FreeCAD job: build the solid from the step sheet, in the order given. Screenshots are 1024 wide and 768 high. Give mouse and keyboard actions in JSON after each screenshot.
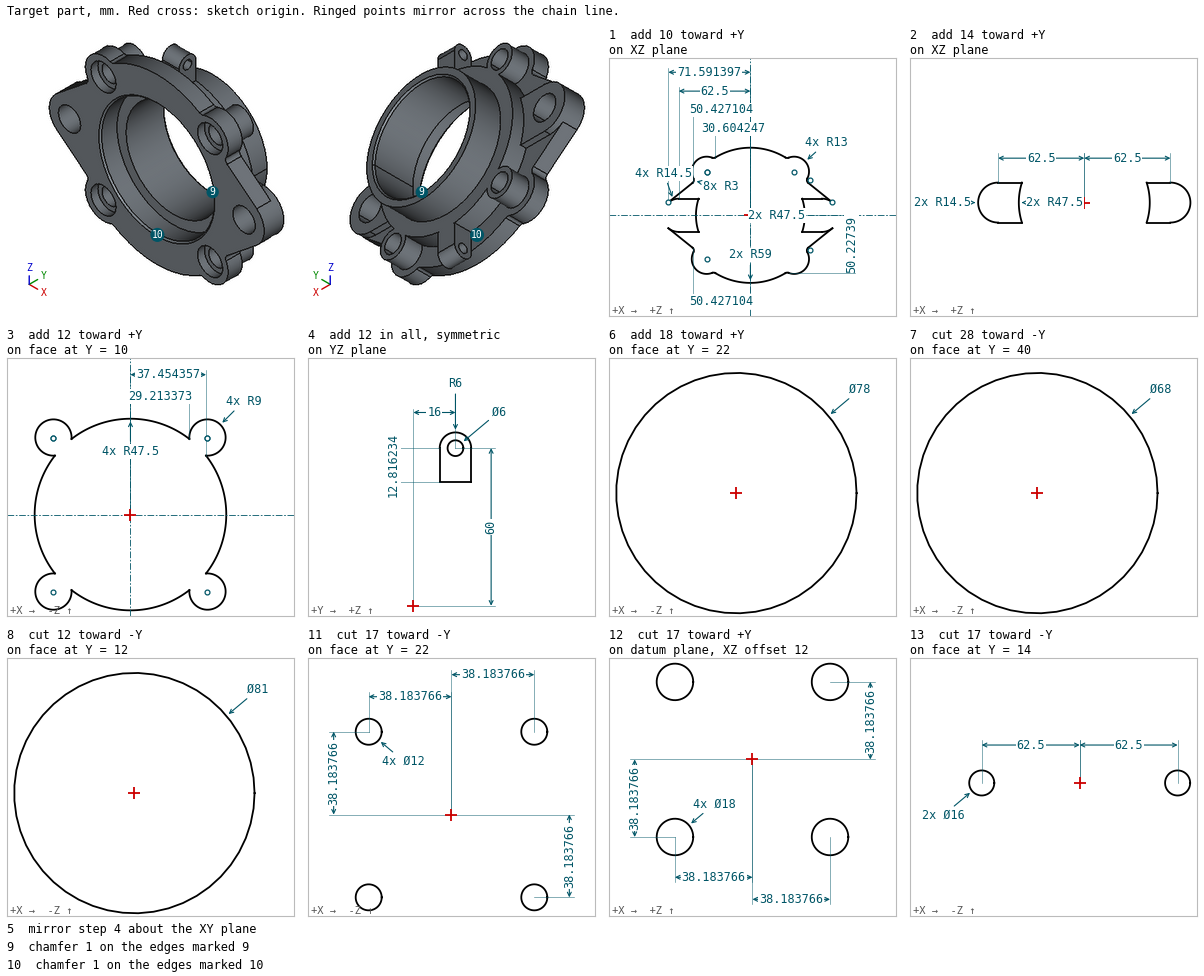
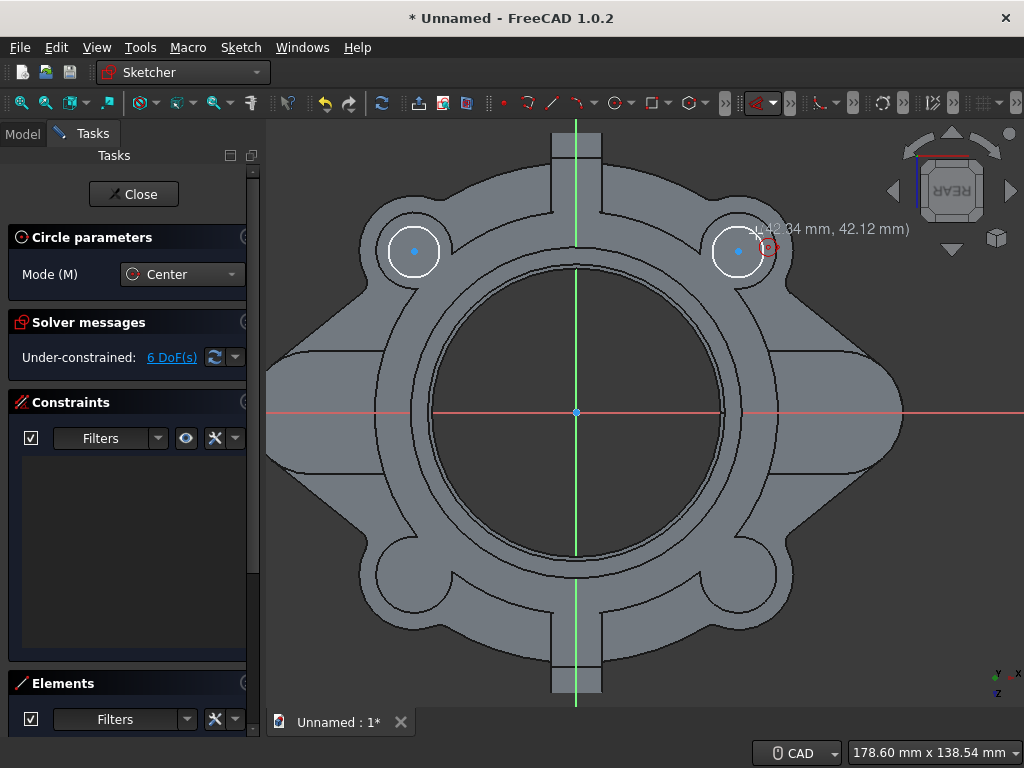
{"action": "left_click", "coordinate": [738, 575]}
{"action": "left_click", "coordinate": [756, 557]}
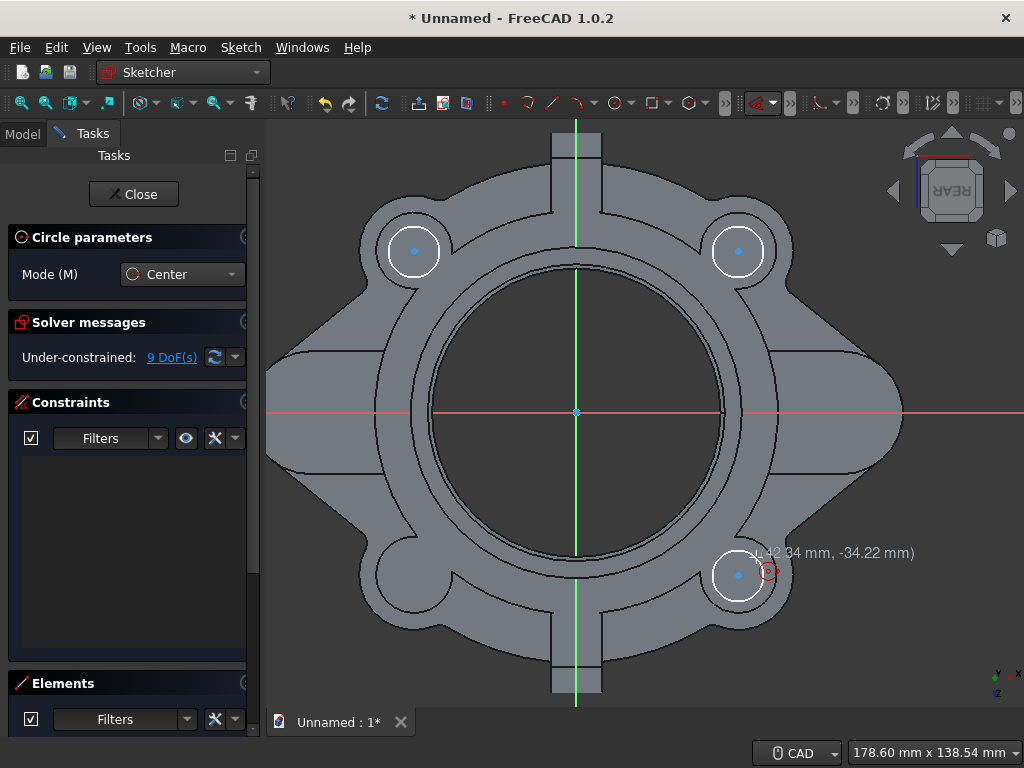
{"action": "left_click", "coordinate": [414, 575]}
{"action": "left_click", "coordinate": [432, 557]}
{"action": "key", "text": "Escape"}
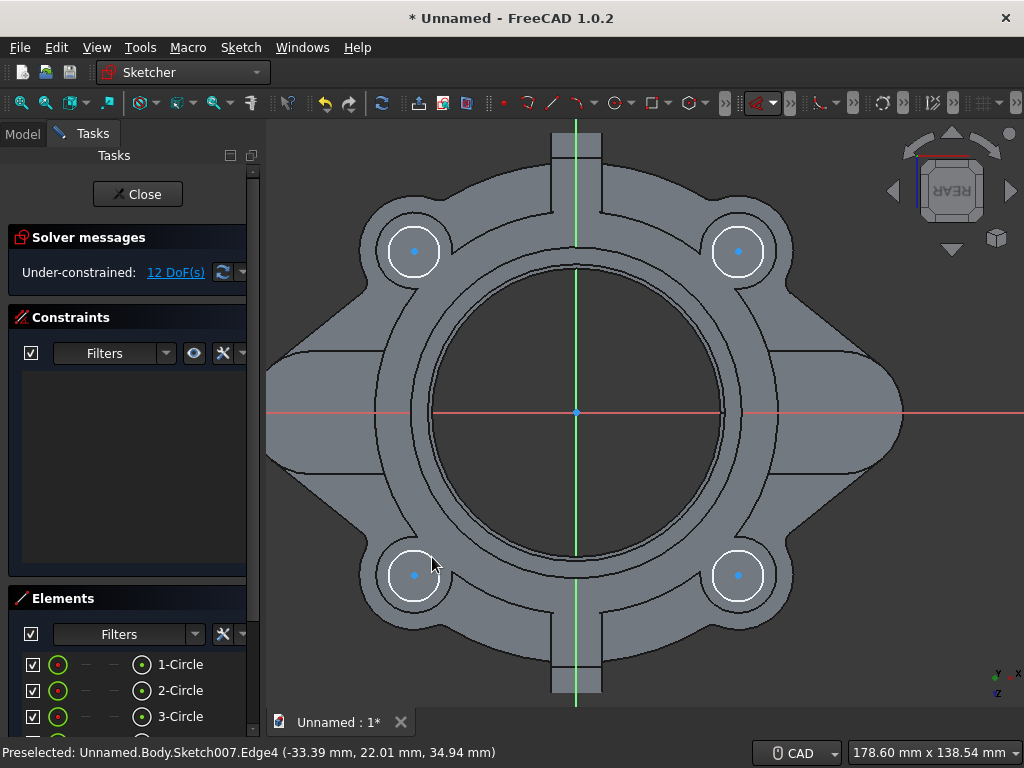
{"action": "left_click", "coordinate": [432, 234]}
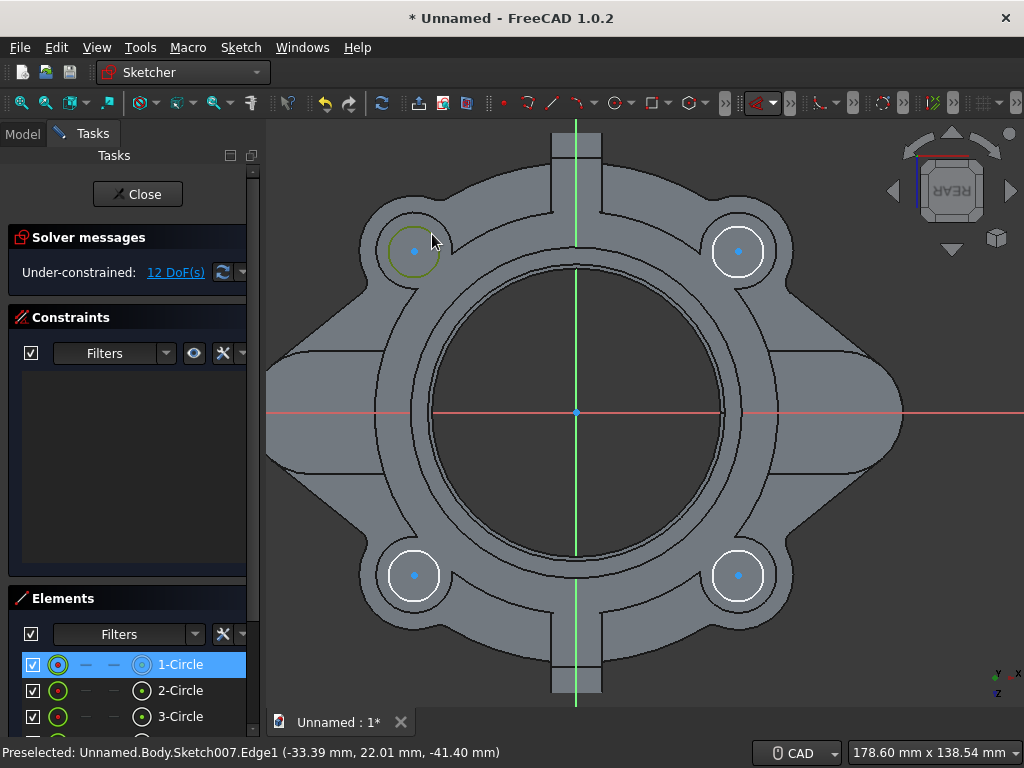
{"action": "left_click", "coordinate": [756, 234]}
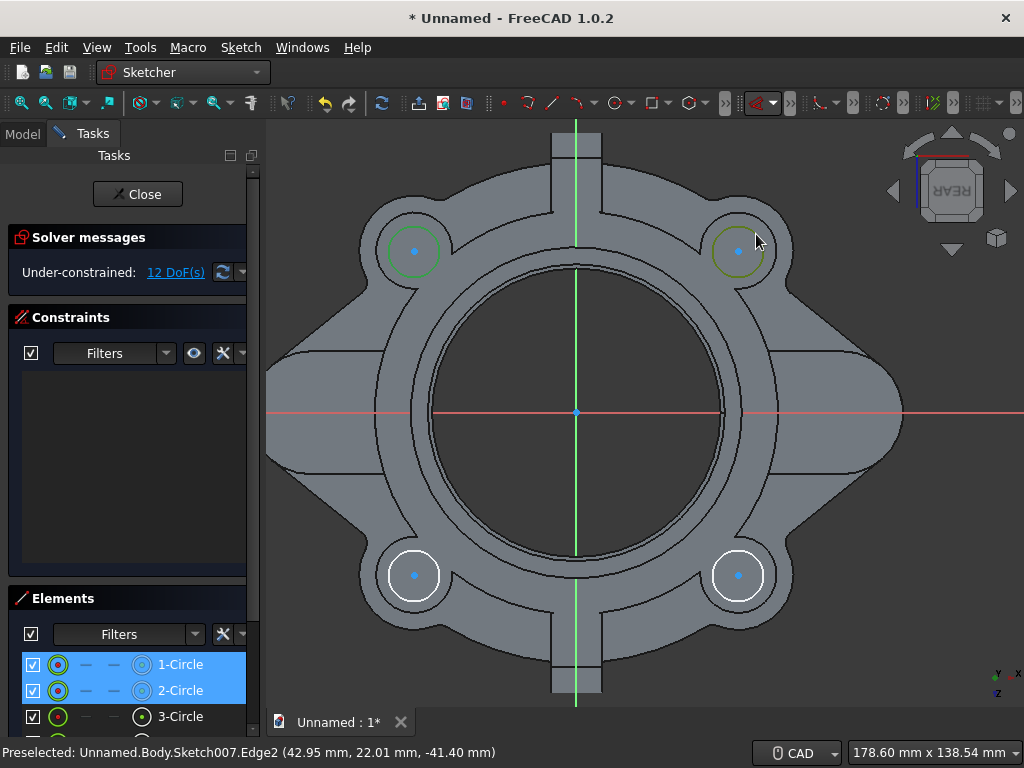
{"action": "left_click", "coordinate": [756, 558]}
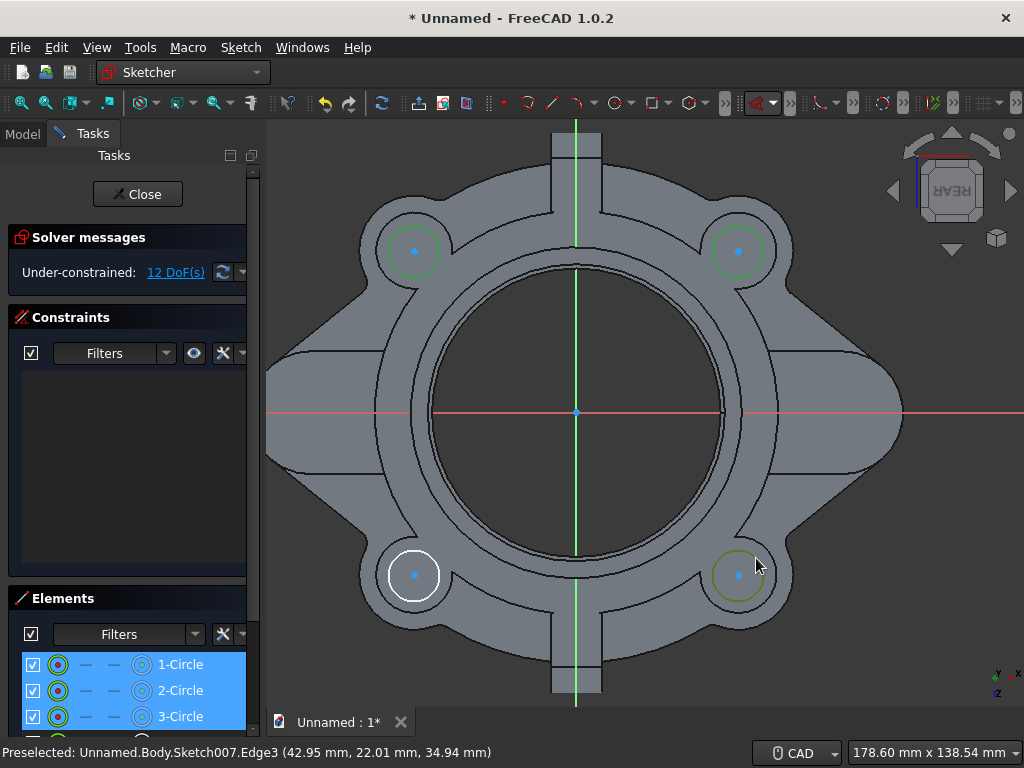
{"action": "left_click", "coordinate": [432, 558]}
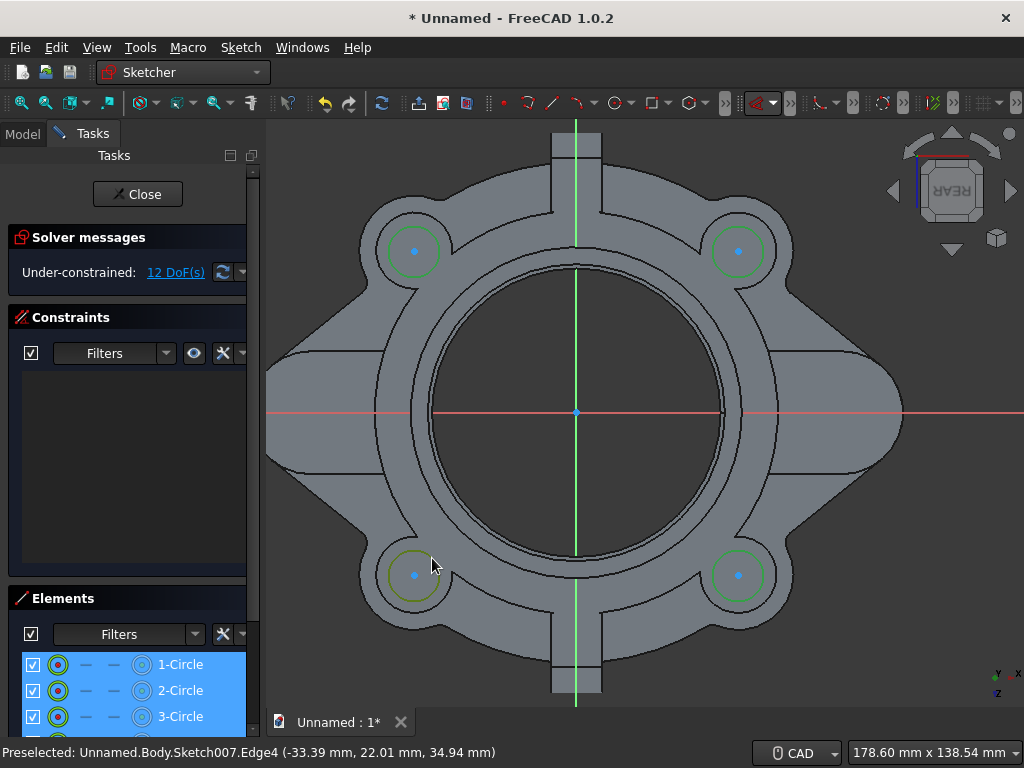
{"action": "key", "text": "e"}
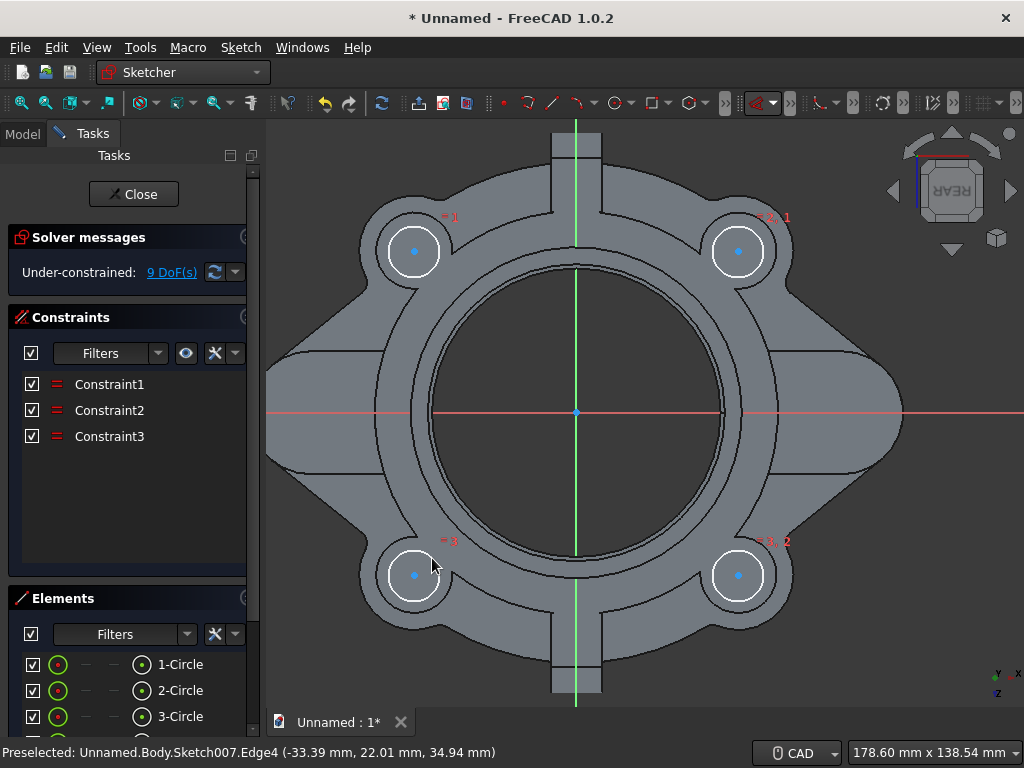
{"action": "left_click", "coordinate": [414, 252]}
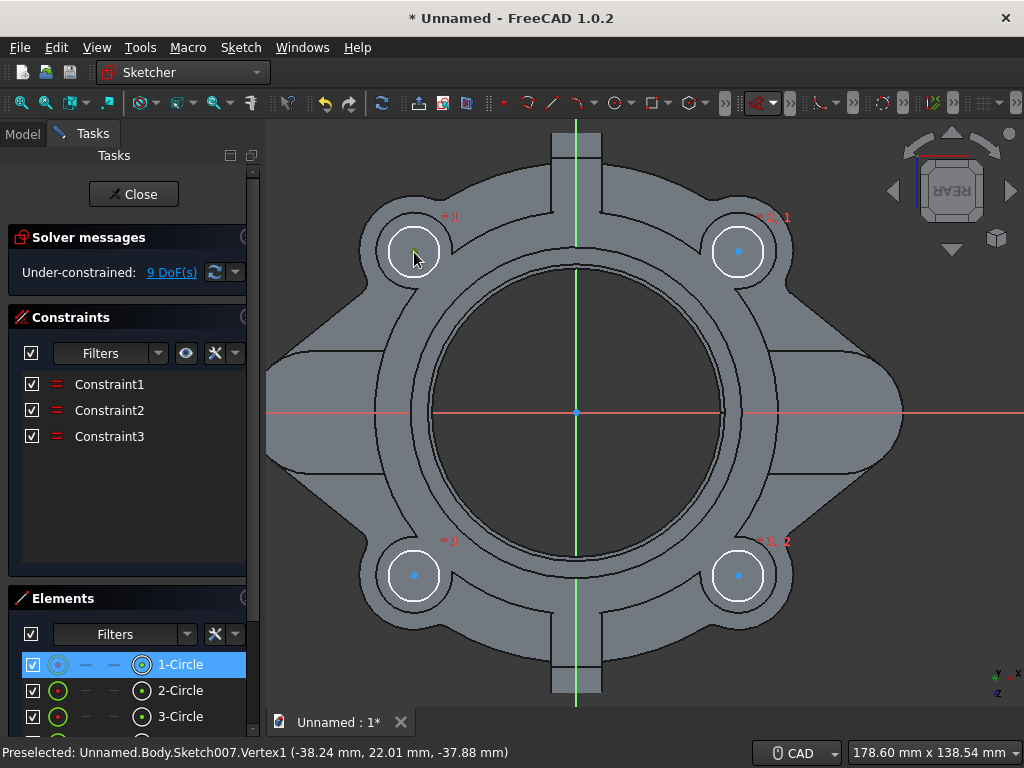
{"action": "left_click", "coordinate": [738, 252]}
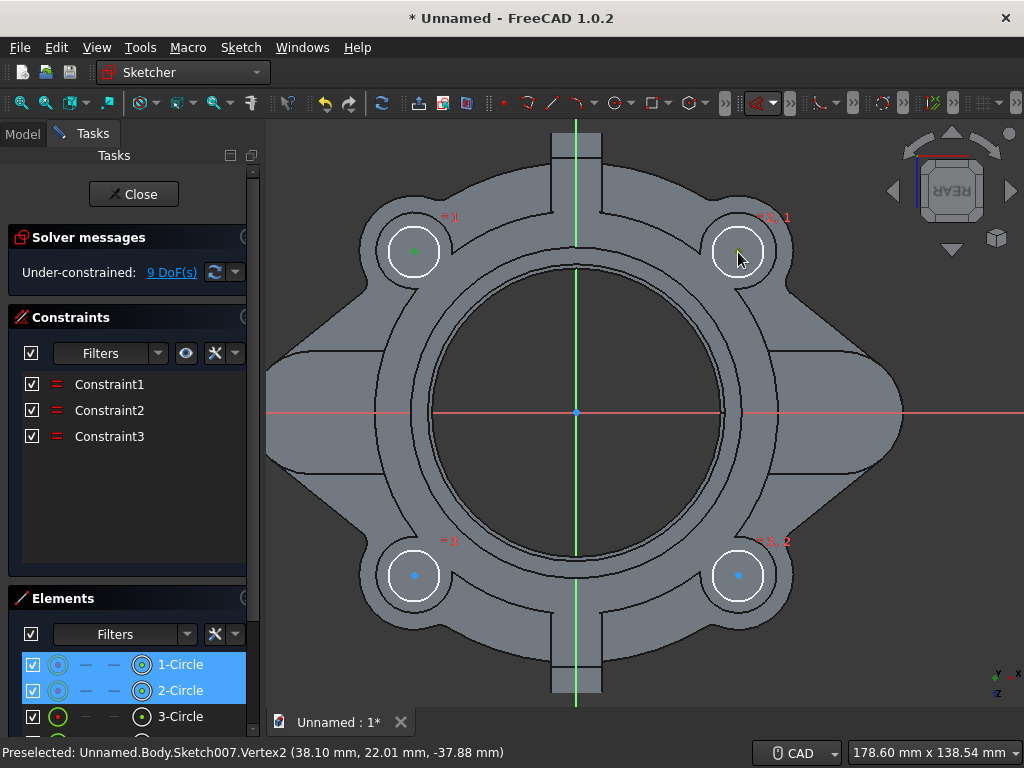
{"action": "key", "text": "h"}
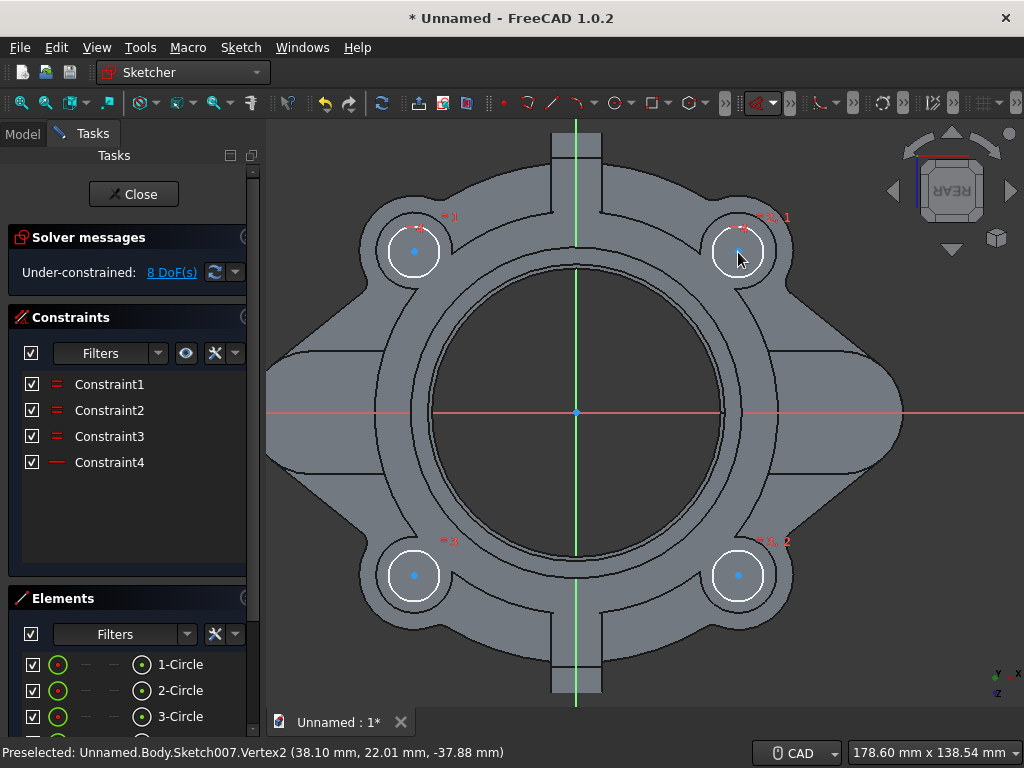
{"action": "left_click", "coordinate": [738, 252]}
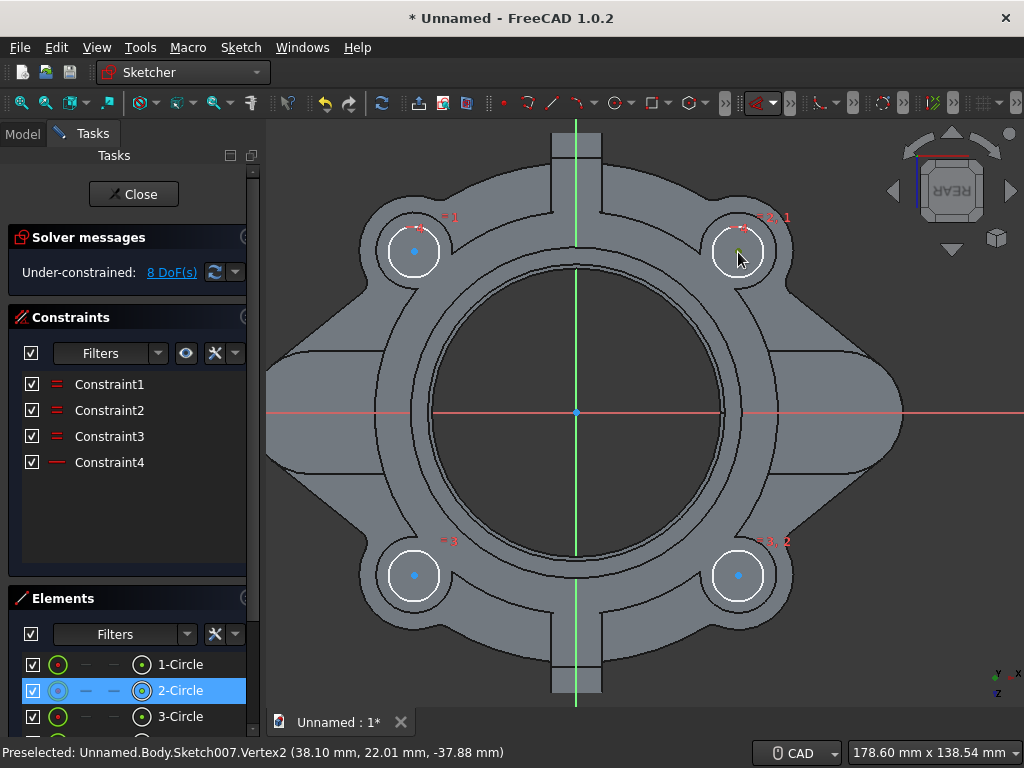
{"action": "left_click", "coordinate": [738, 576]}